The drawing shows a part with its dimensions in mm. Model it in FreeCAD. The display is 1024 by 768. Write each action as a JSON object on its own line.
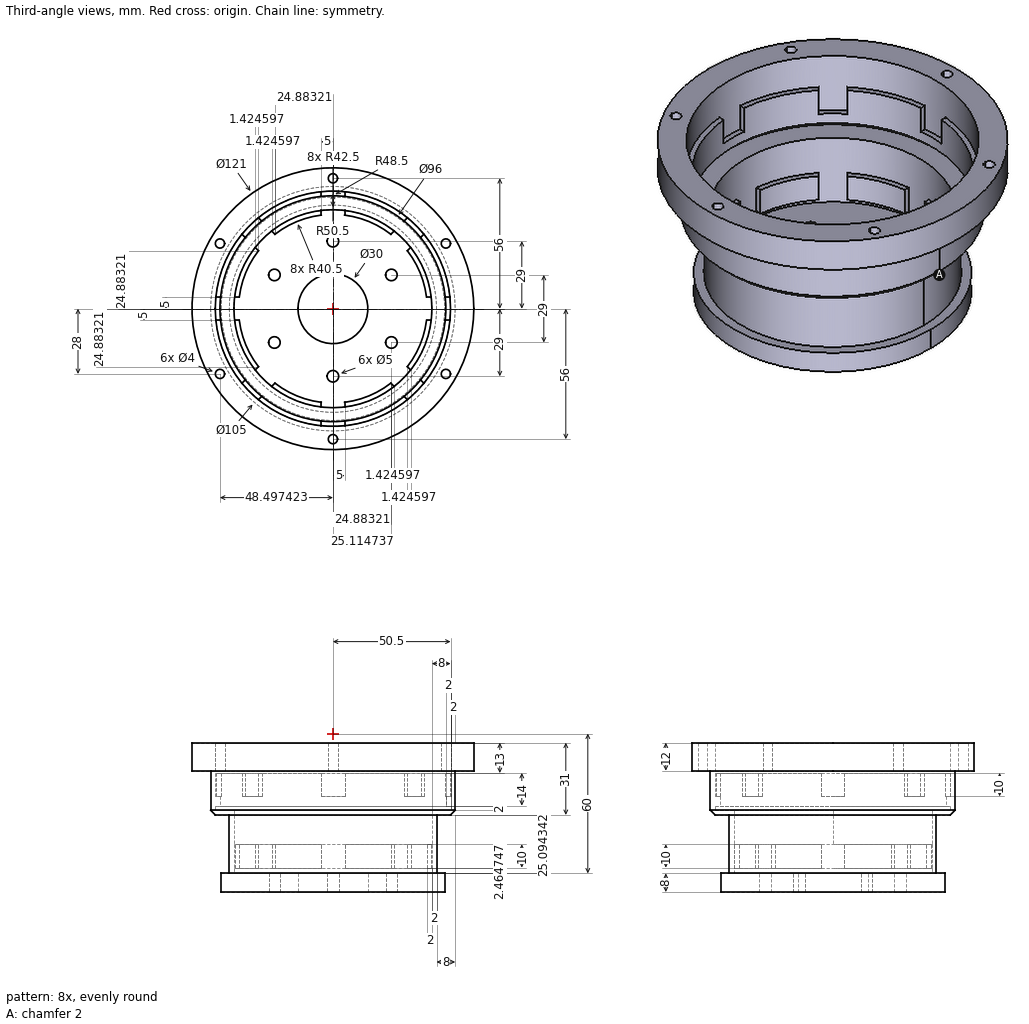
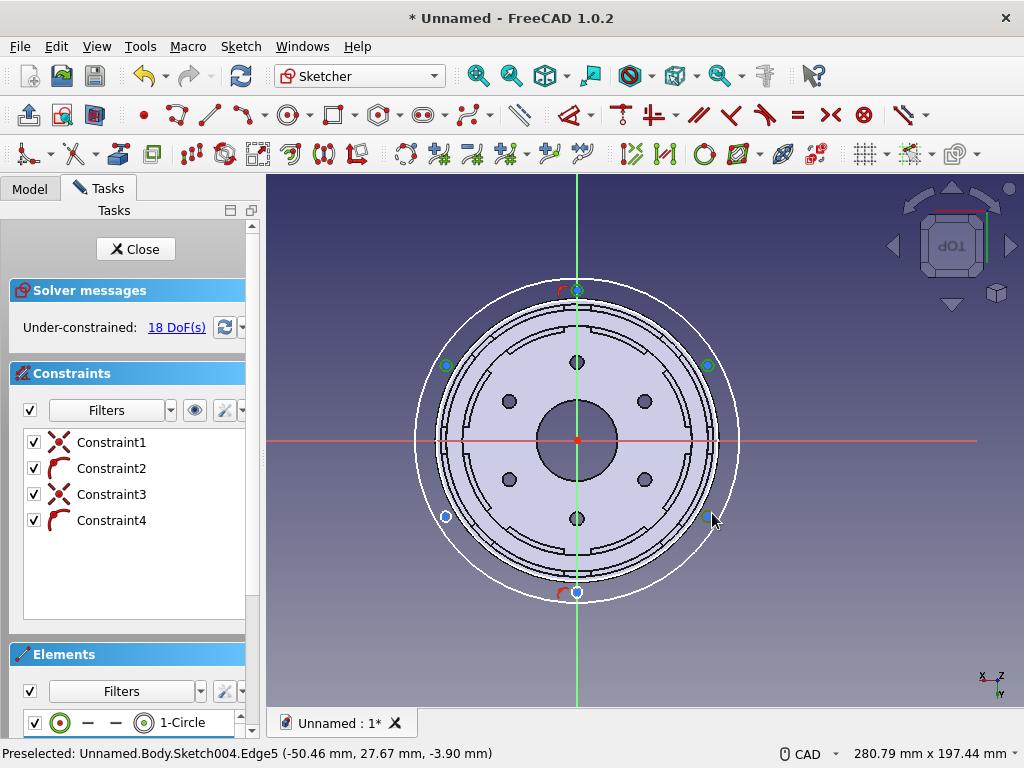
{"action": "scroll", "coordinate": [450, 513], "scroll_direction": "up", "scroll_amount": 5}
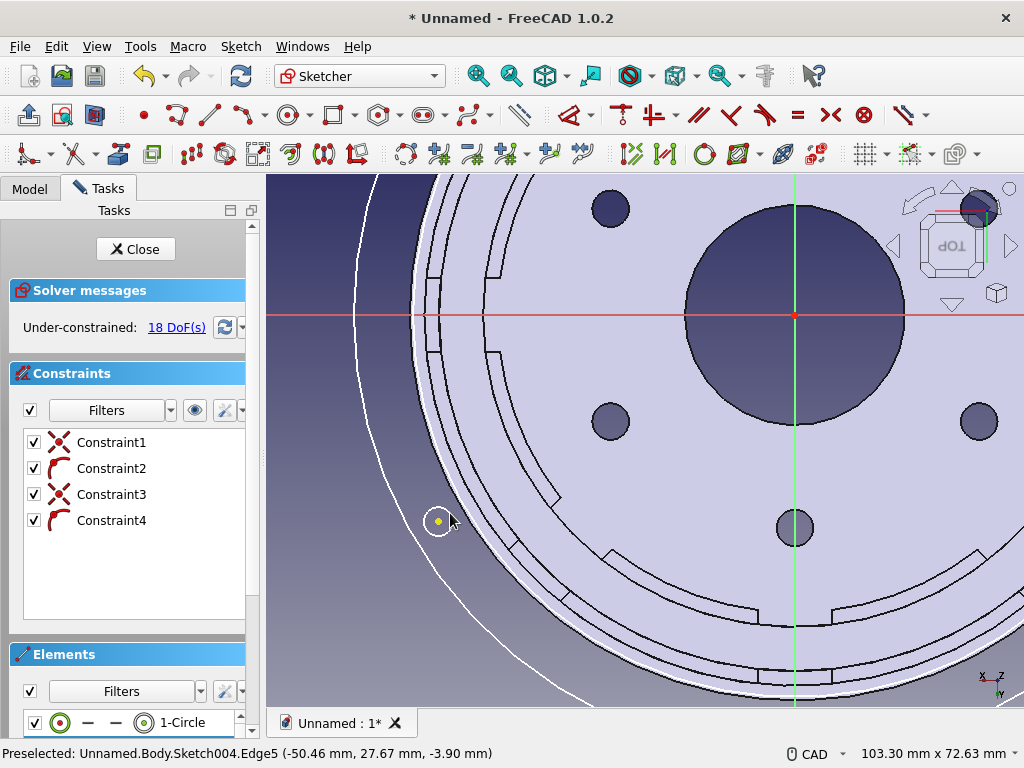
{"action": "left_click", "coordinate": [448, 511]}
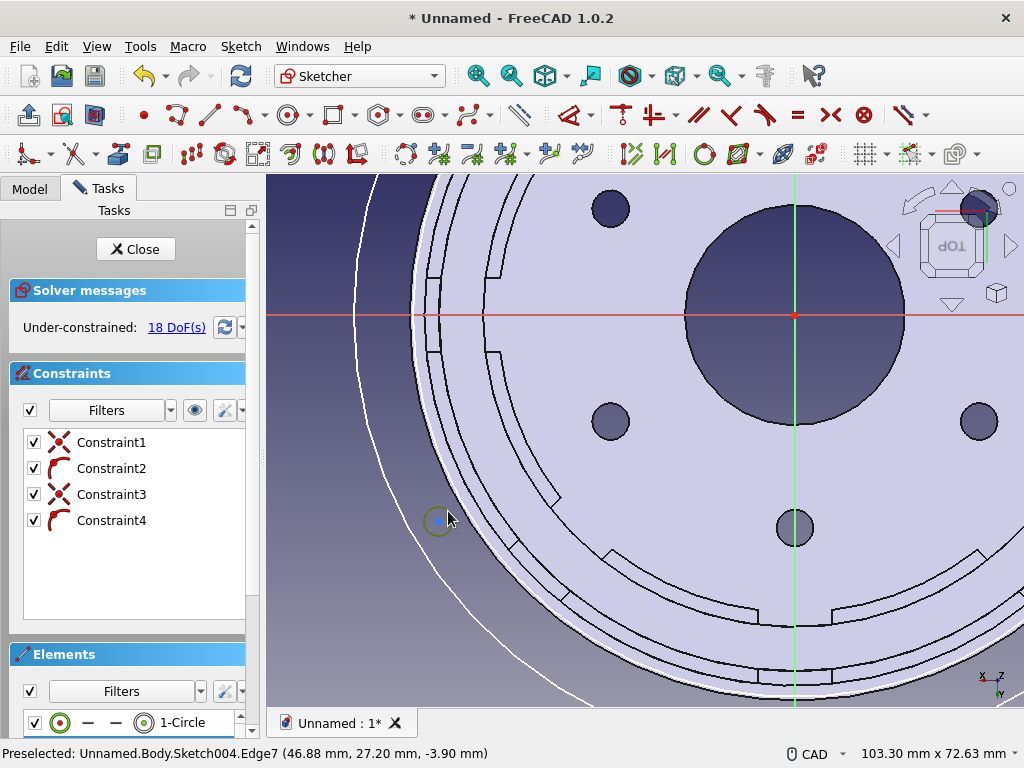
{"action": "scroll", "coordinate": [449, 513], "scroll_direction": "down", "scroll_amount": 5}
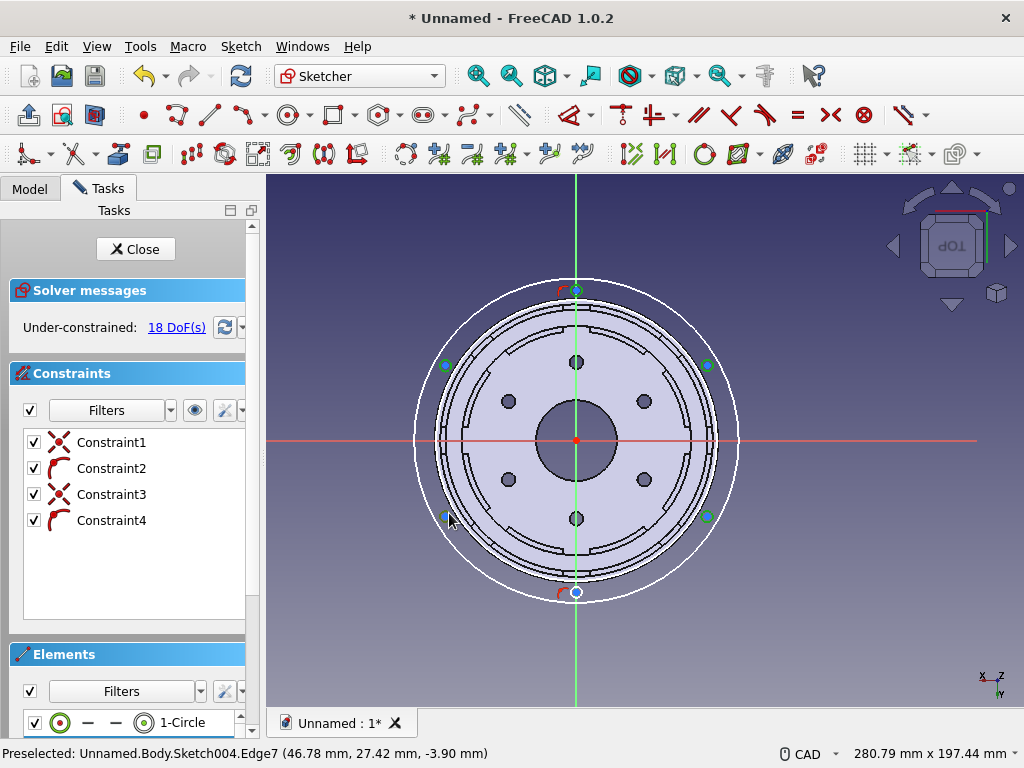
{"action": "scroll", "coordinate": [580, 588], "scroll_direction": "up", "scroll_amount": 7}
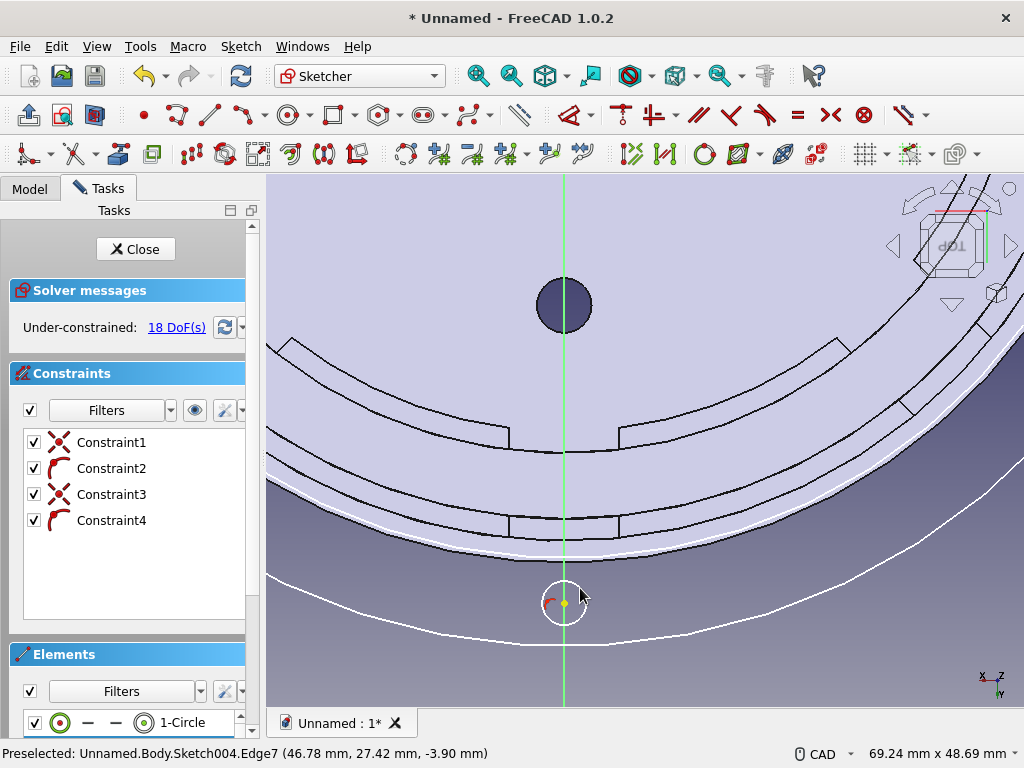
{"action": "left_click", "coordinate": [580, 588]}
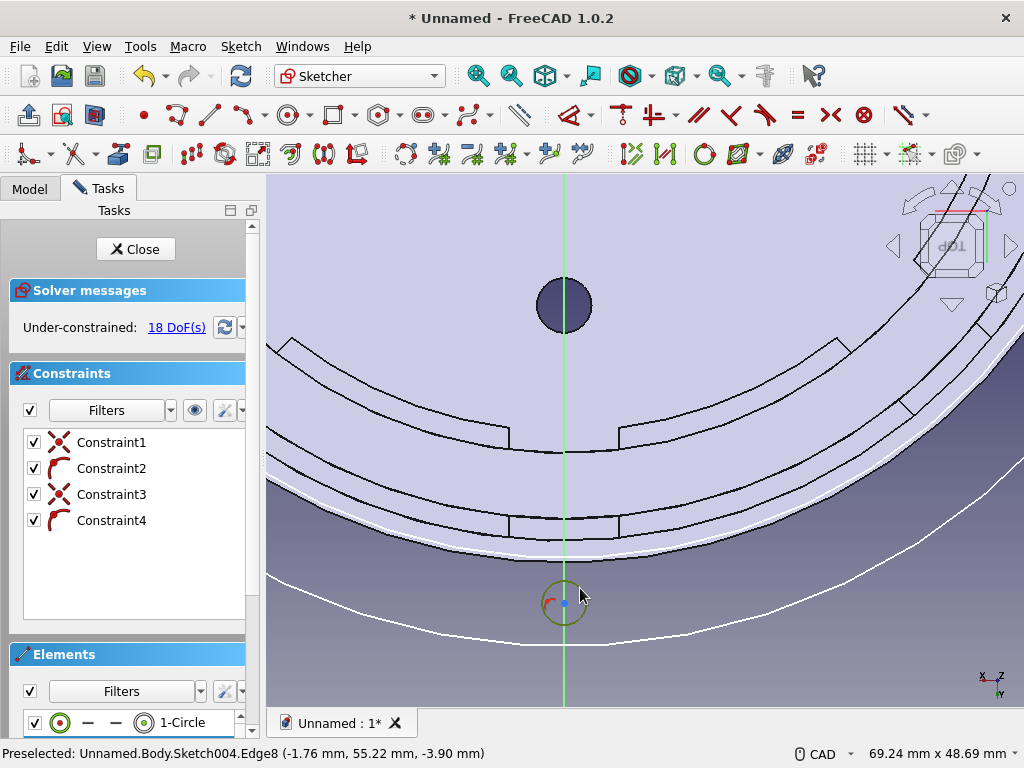
{"action": "key", "text": "e"}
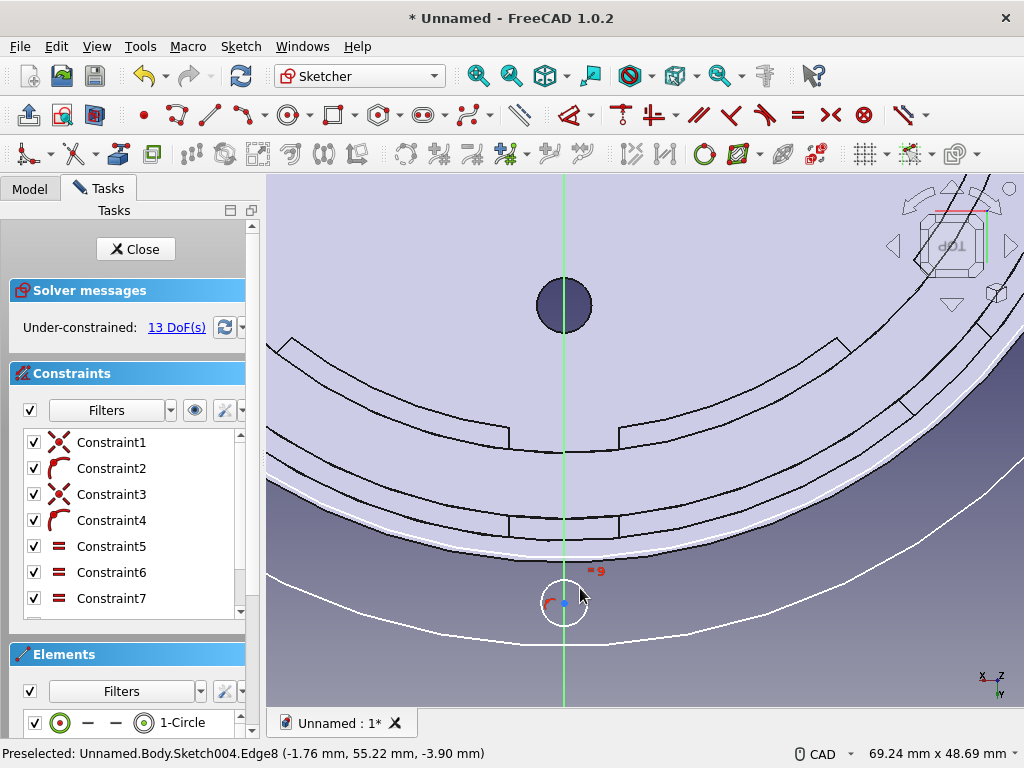
{"action": "scroll", "coordinate": [581, 589], "scroll_direction": "down", "scroll_amount": 7}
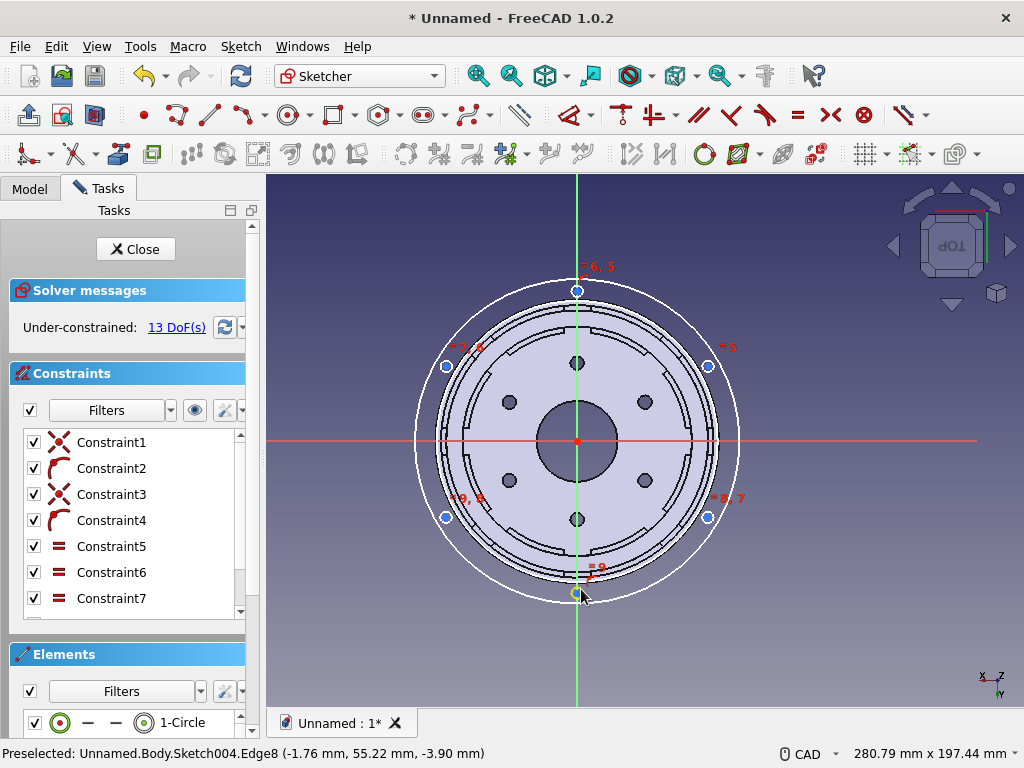
{"action": "left_click", "coordinate": [708, 366]}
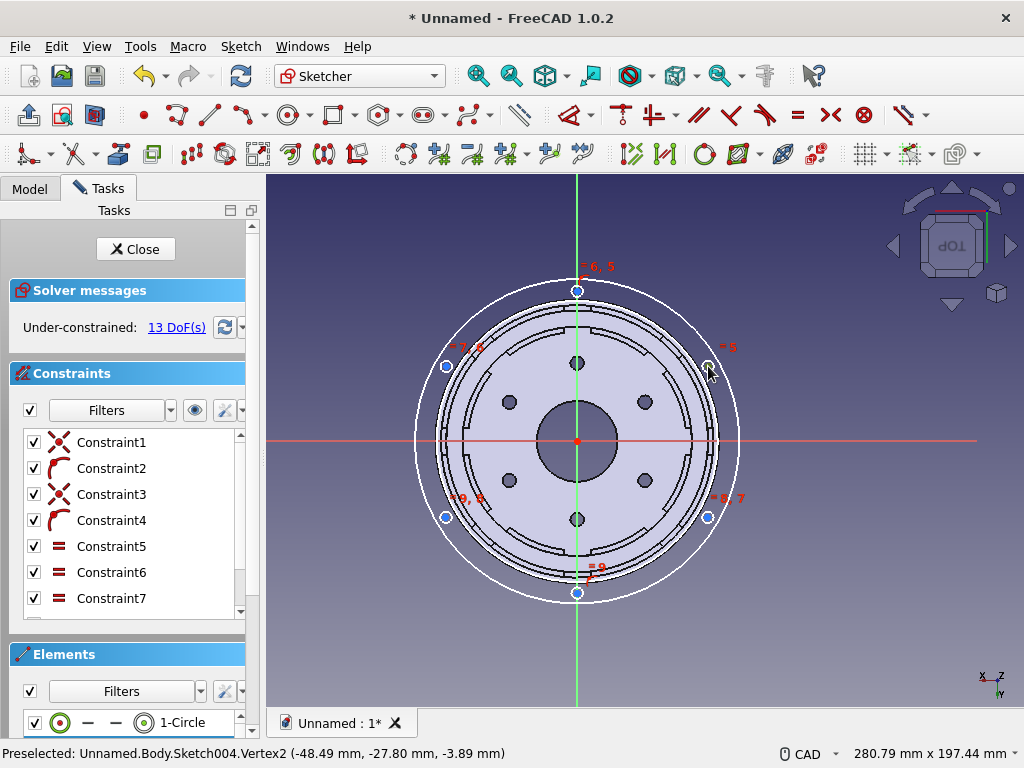
{"action": "left_click", "coordinate": [446, 367]}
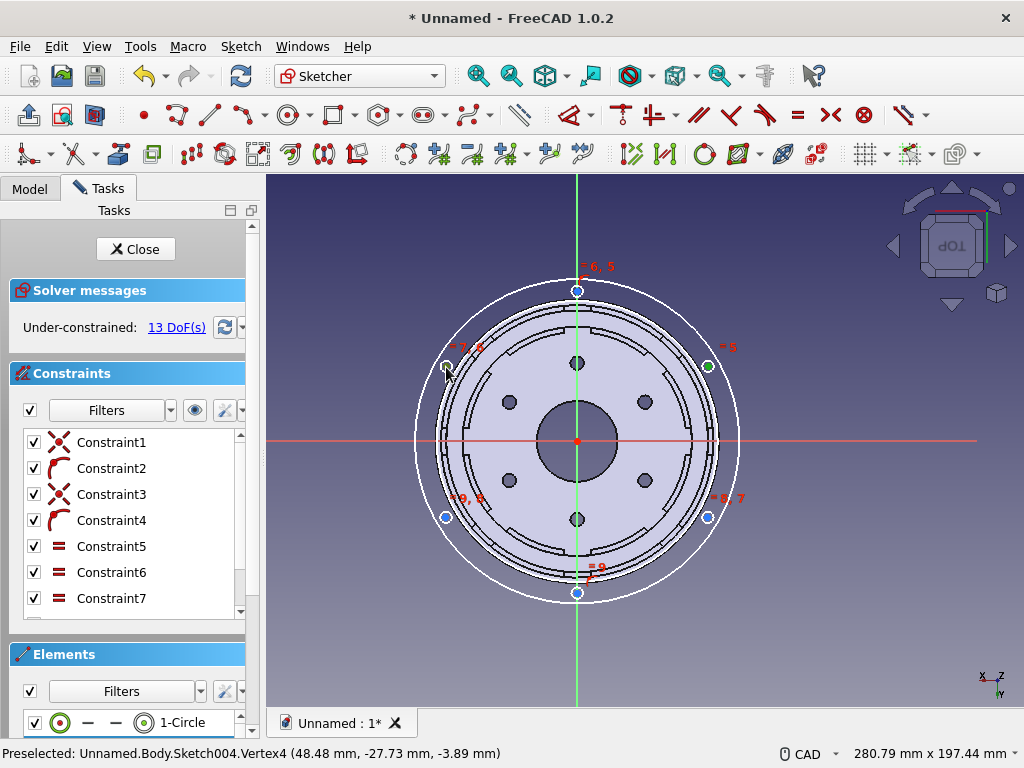
{"action": "left_click", "coordinate": [577, 645]}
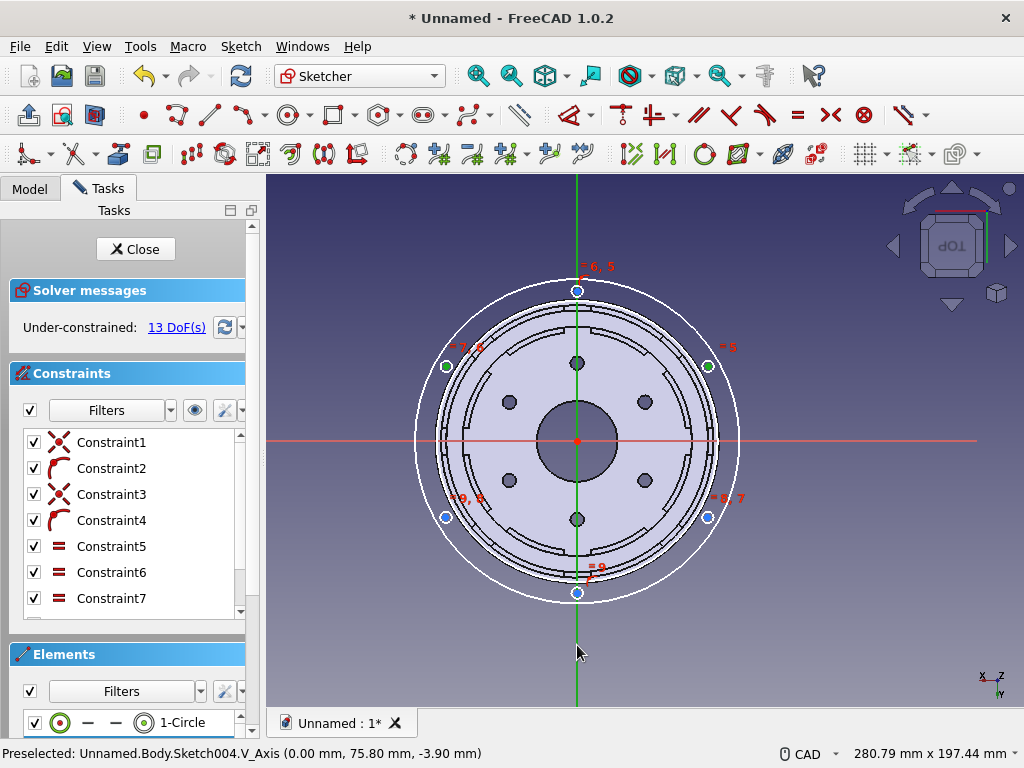
{"action": "key", "text": "s"}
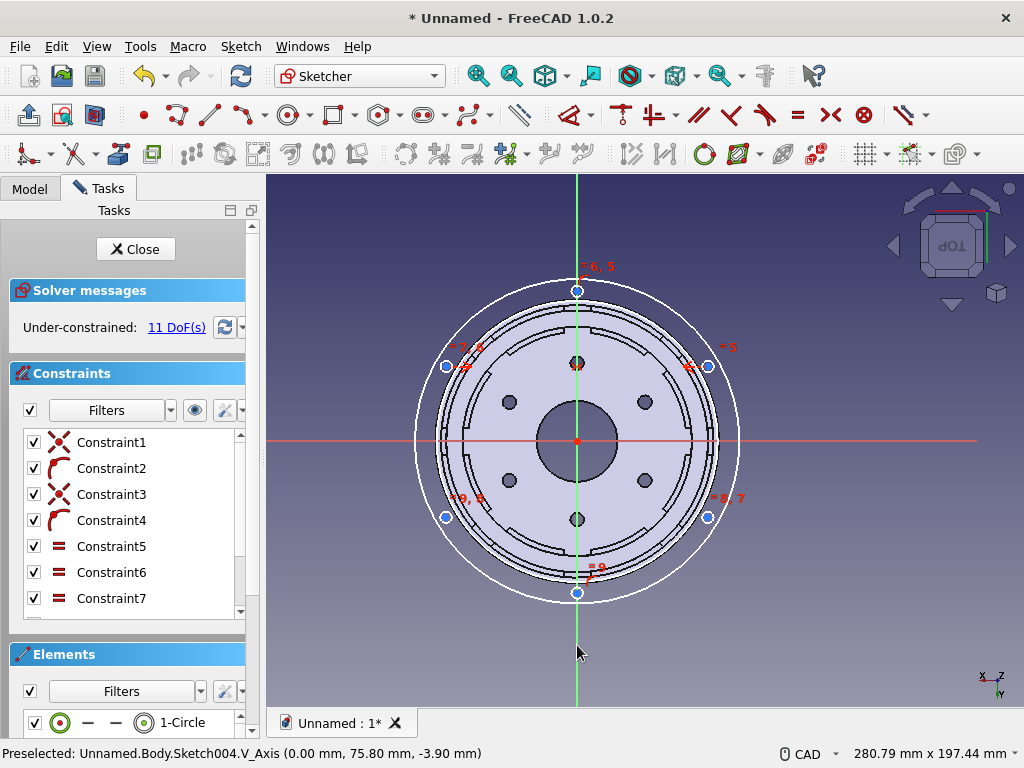
{"action": "left_click", "coordinate": [708, 367]}